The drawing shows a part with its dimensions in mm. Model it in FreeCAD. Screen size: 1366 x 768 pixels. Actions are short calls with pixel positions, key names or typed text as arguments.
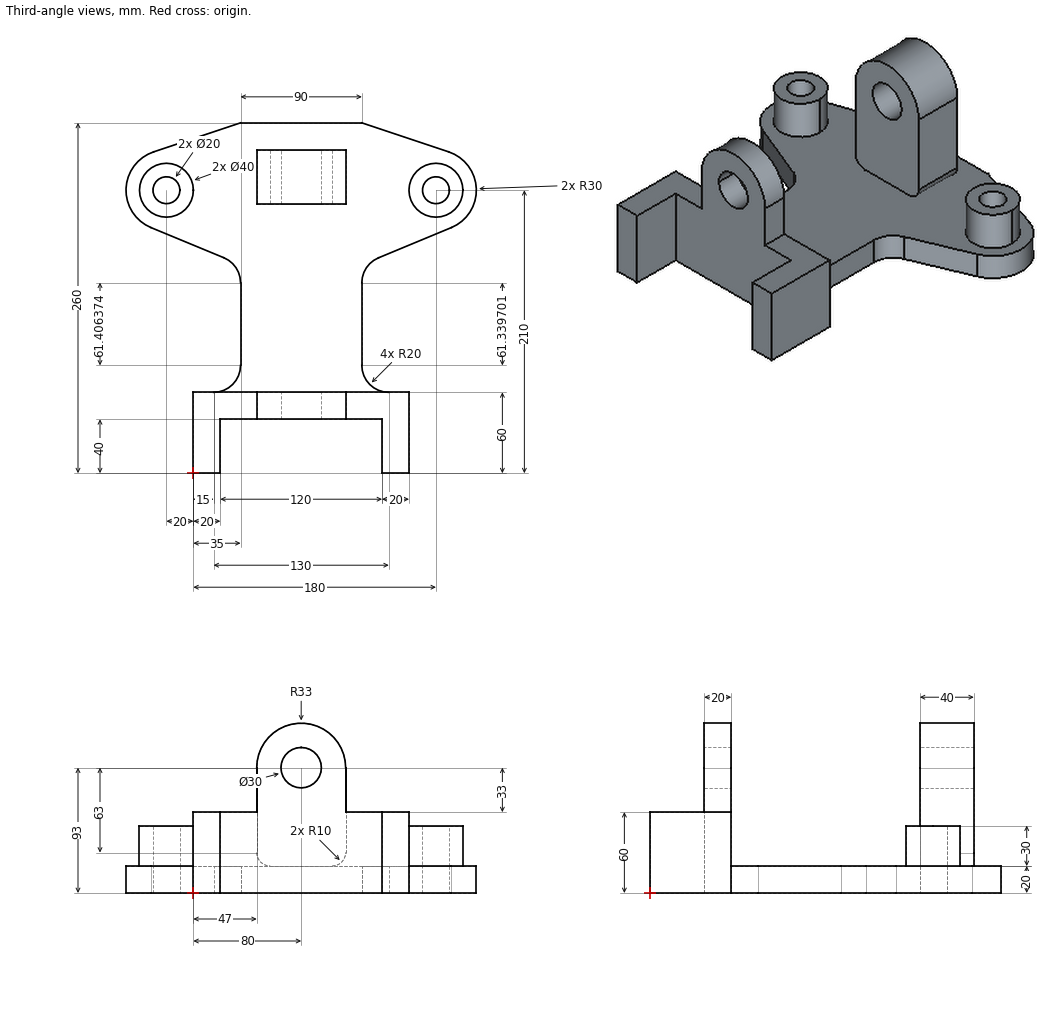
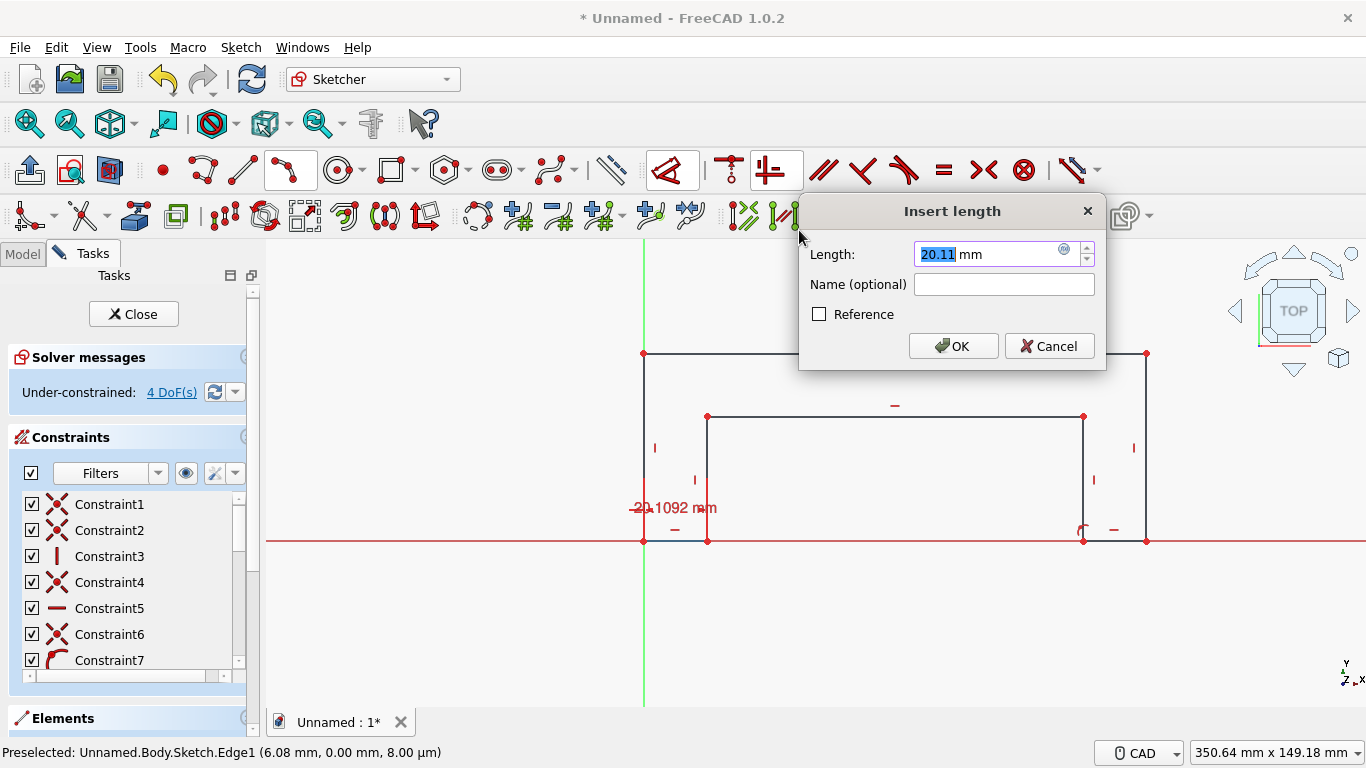
text(20)
key(Return)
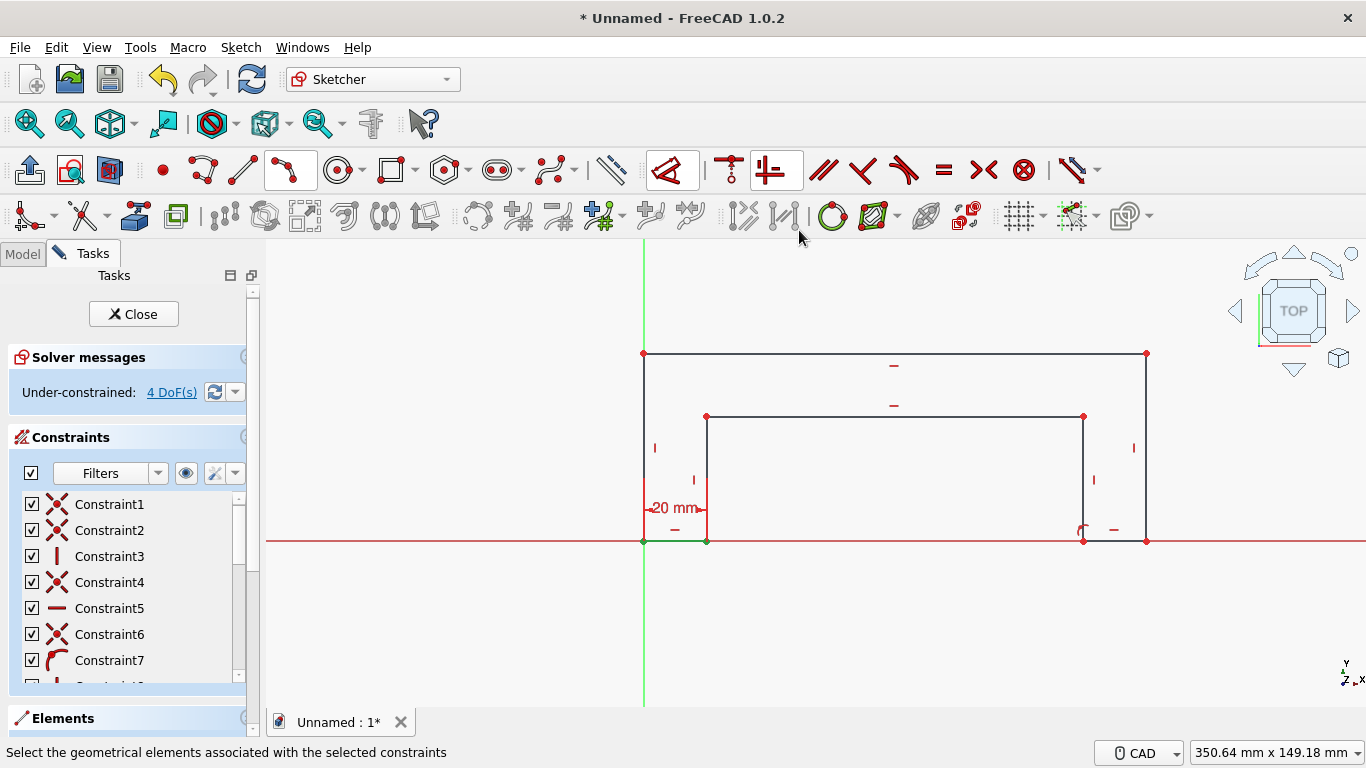
click(707, 504)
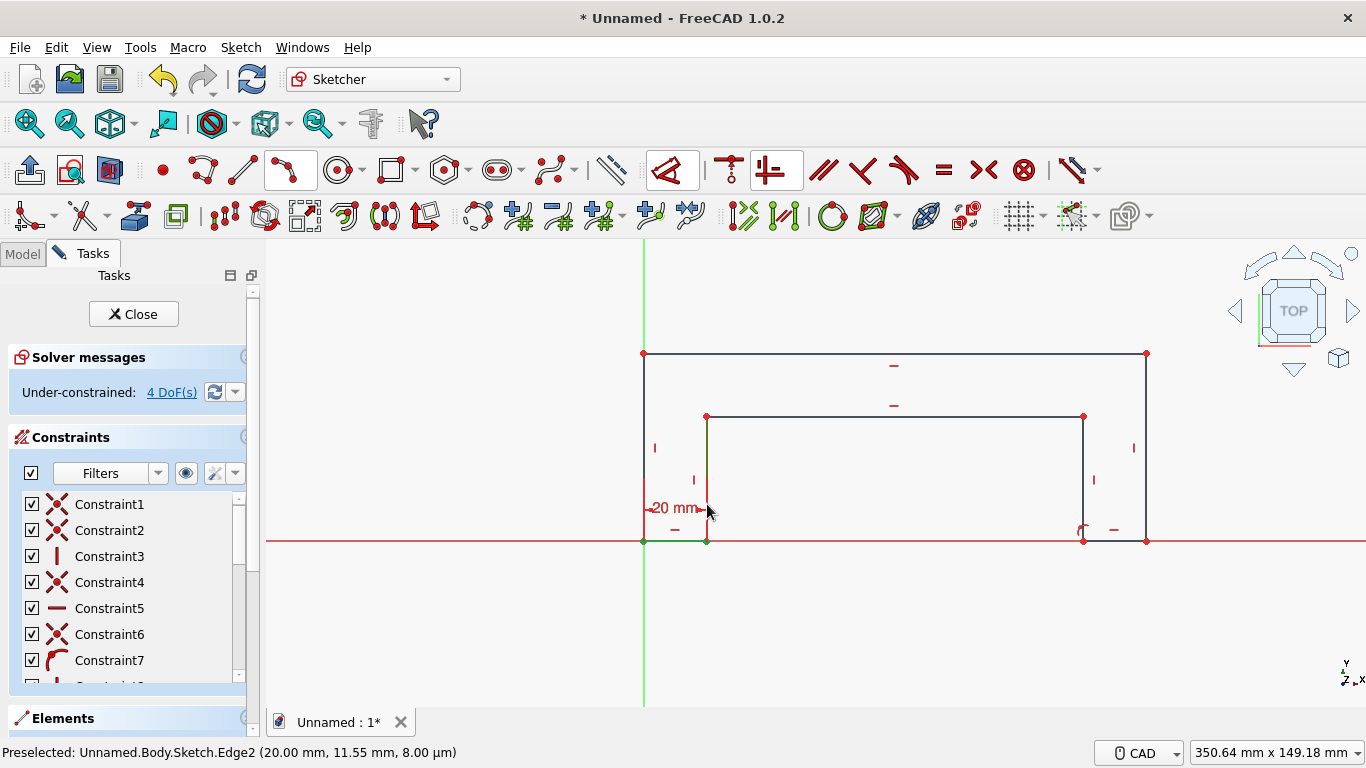
click(694, 170)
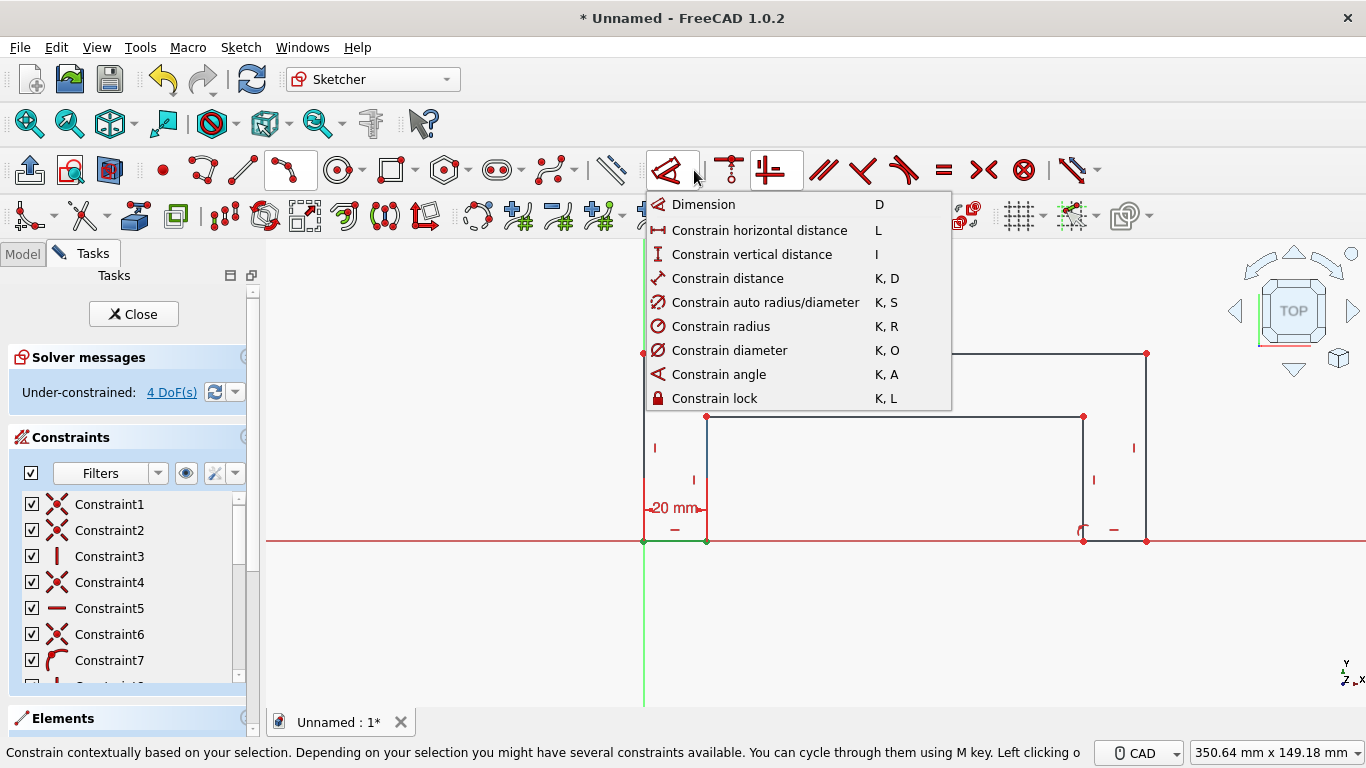
click(799, 254)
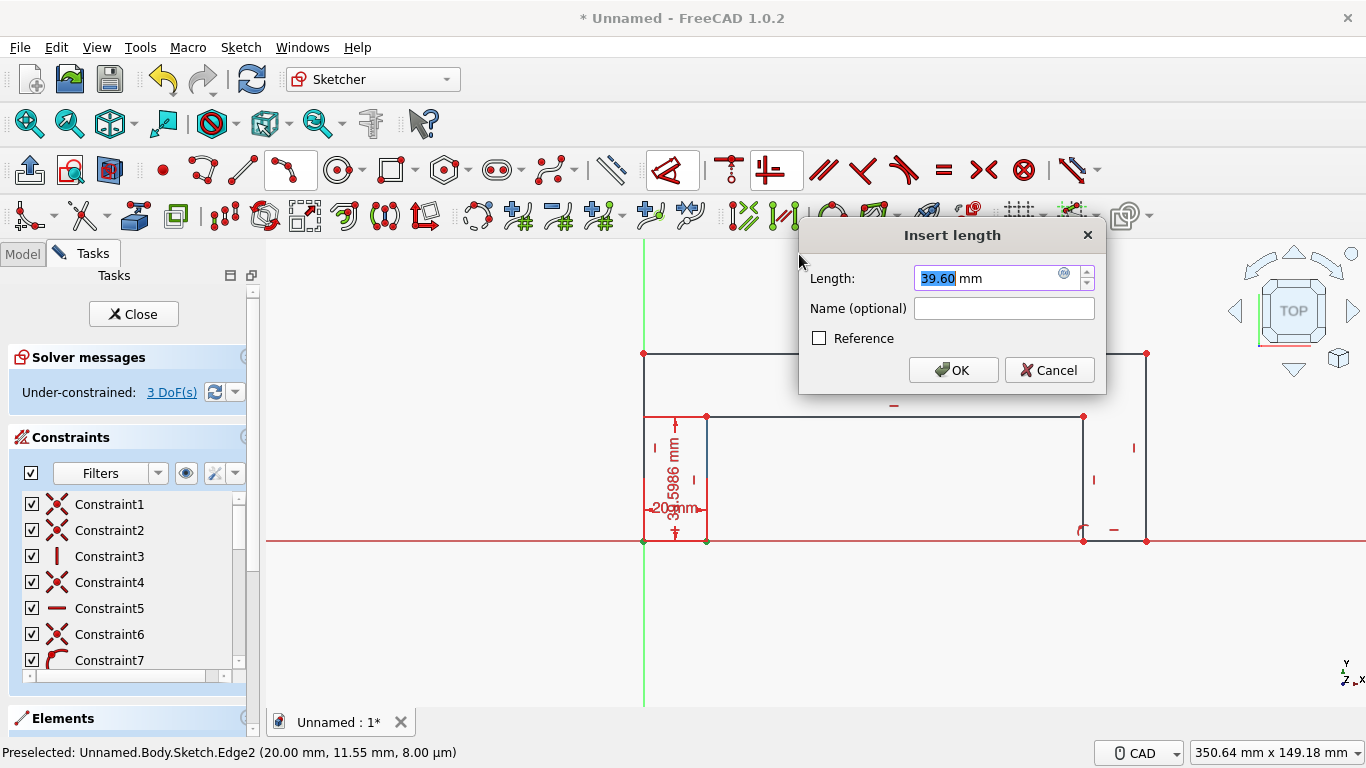
text(40)
key(Return)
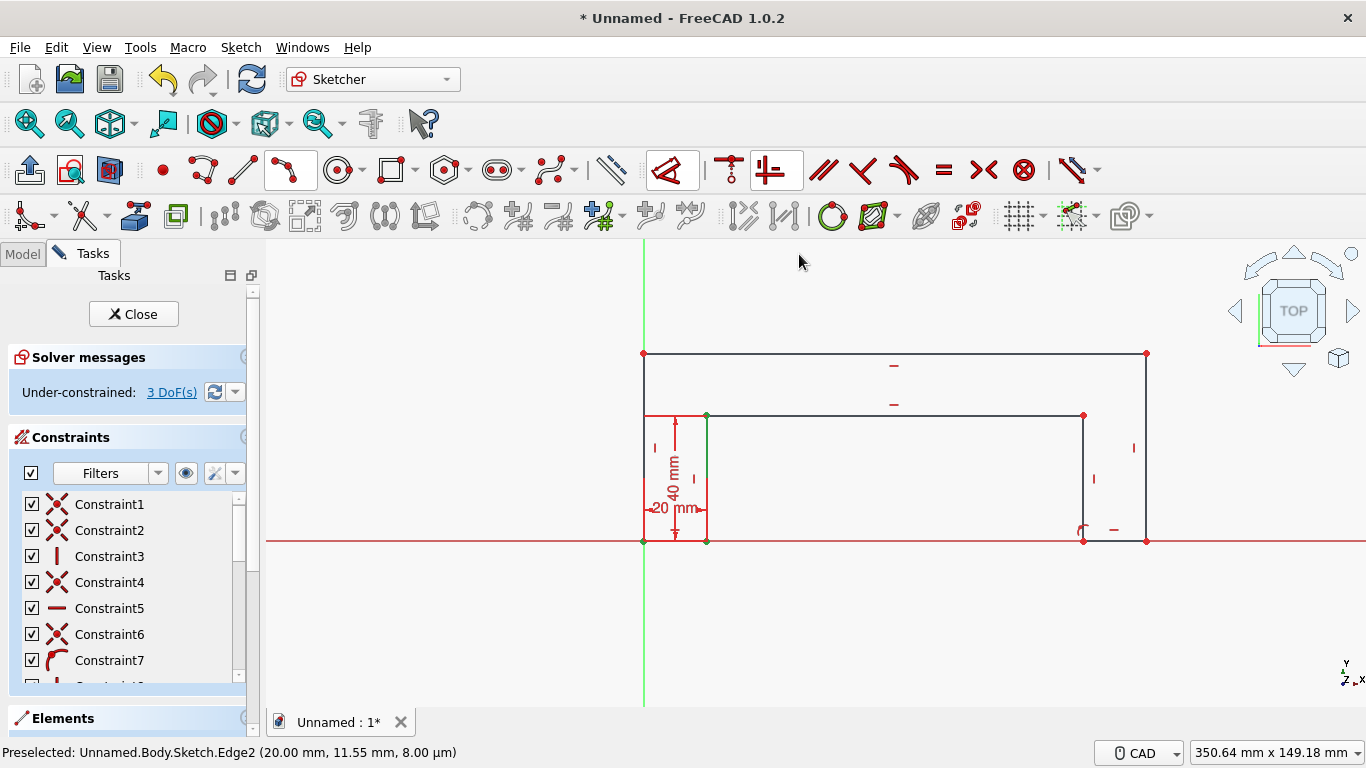
click(1102, 541)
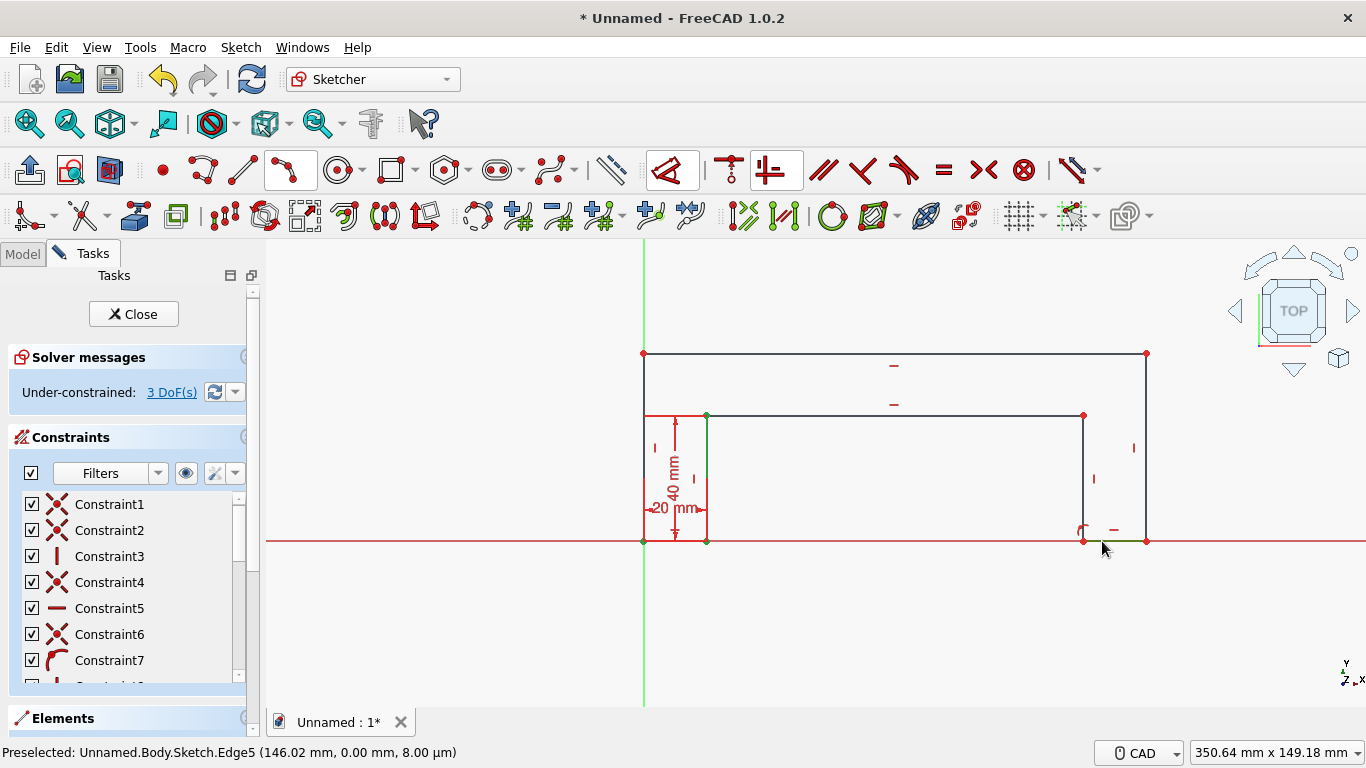
key(l)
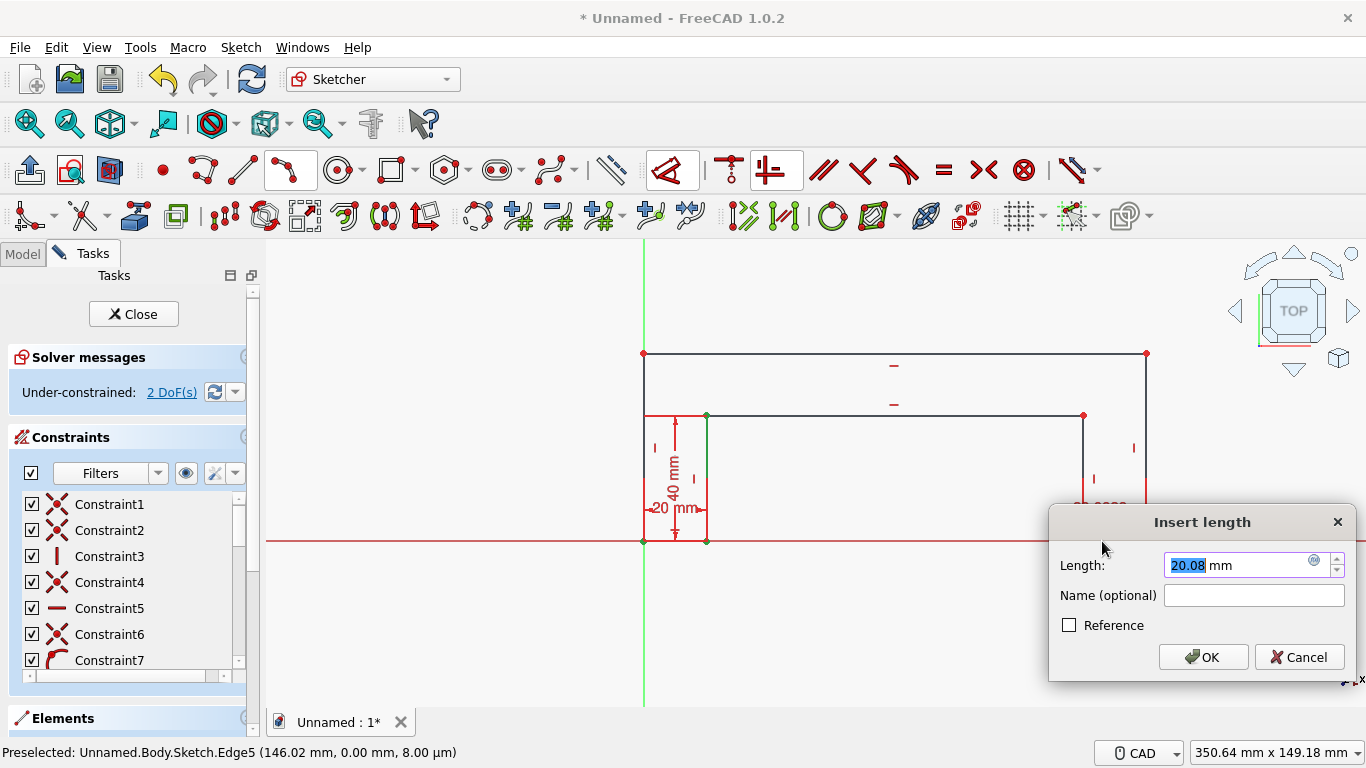
text(20)
key(Return)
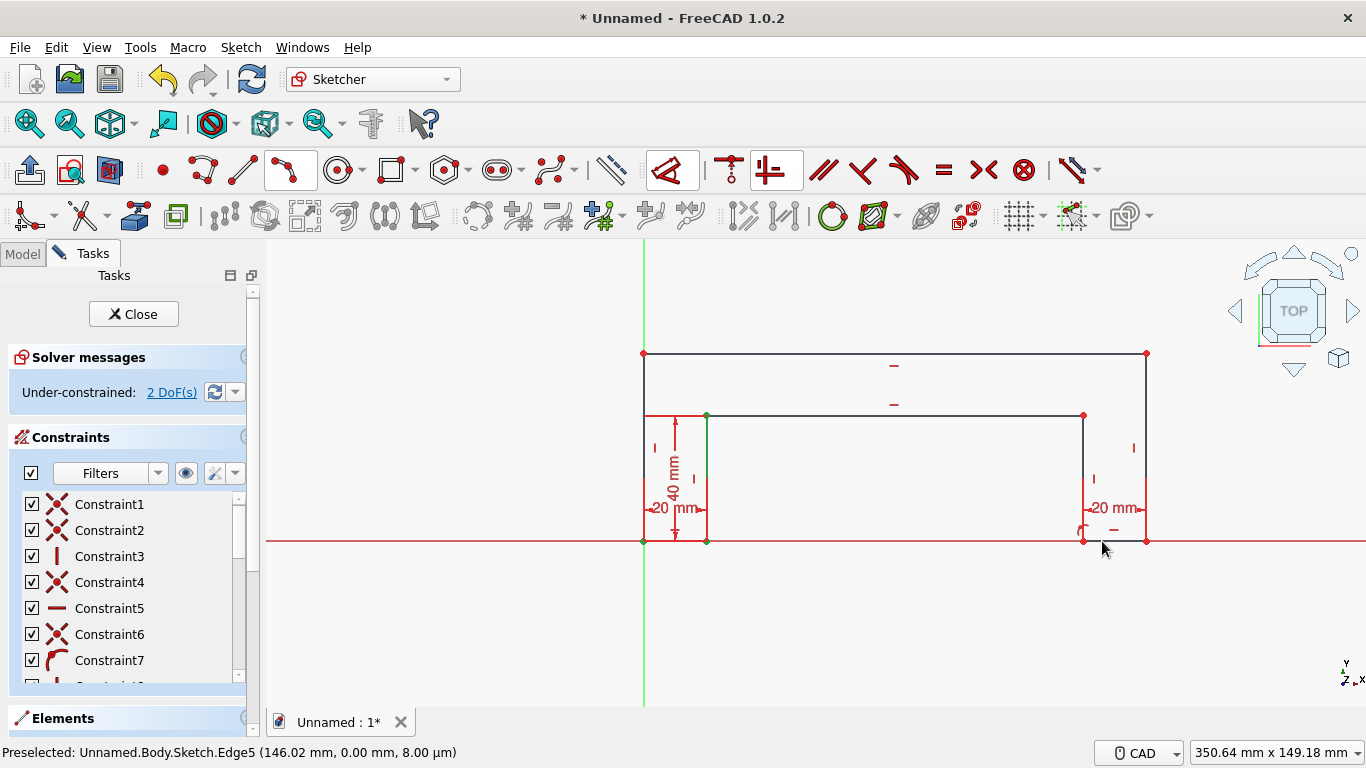
click(1146, 485)